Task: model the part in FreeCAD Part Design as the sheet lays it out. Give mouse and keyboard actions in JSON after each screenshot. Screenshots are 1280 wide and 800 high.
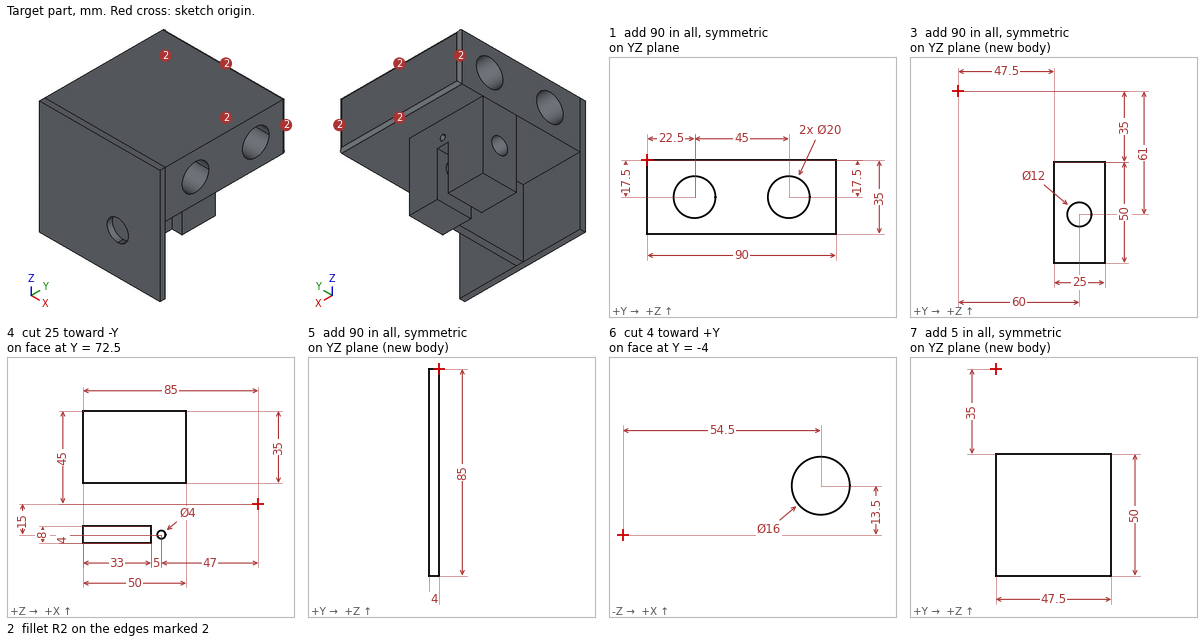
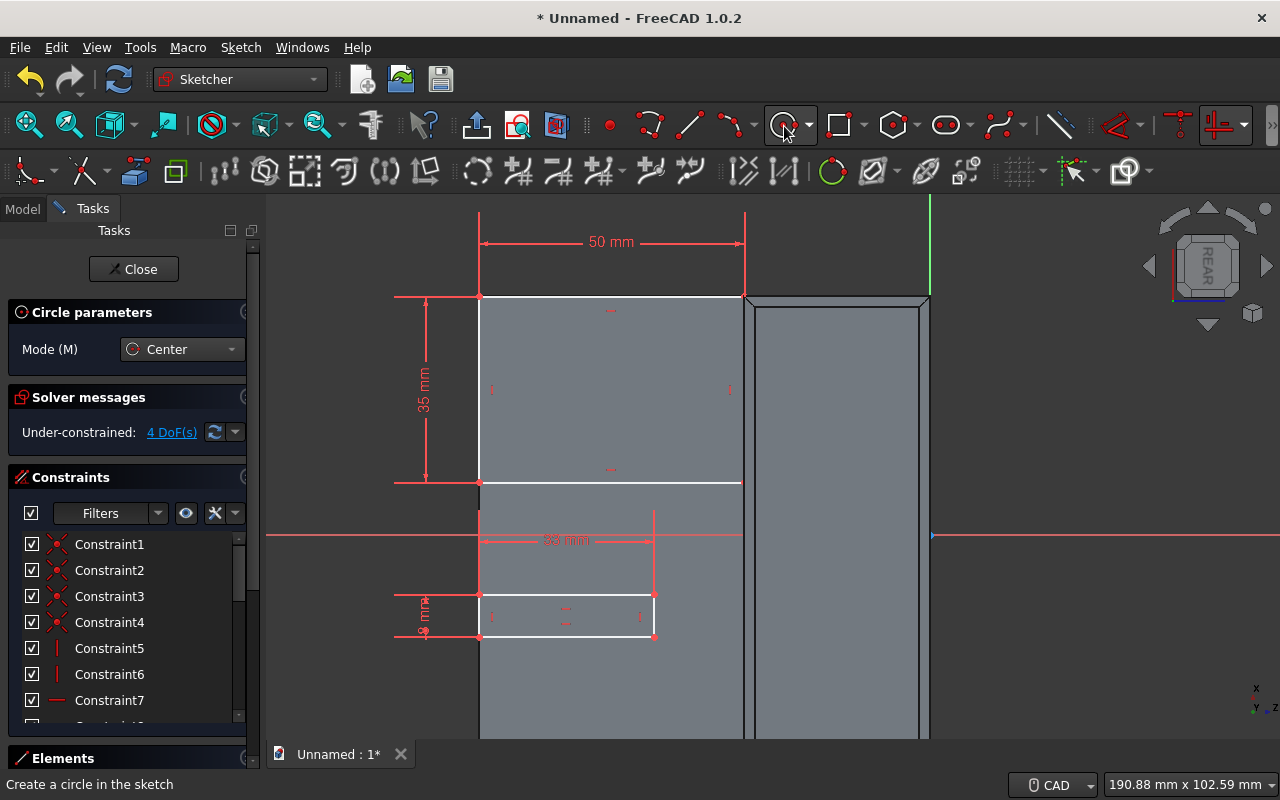
{"action": "scroll", "coordinate": [680, 615], "scroll_direction": "up", "scroll_amount": 4}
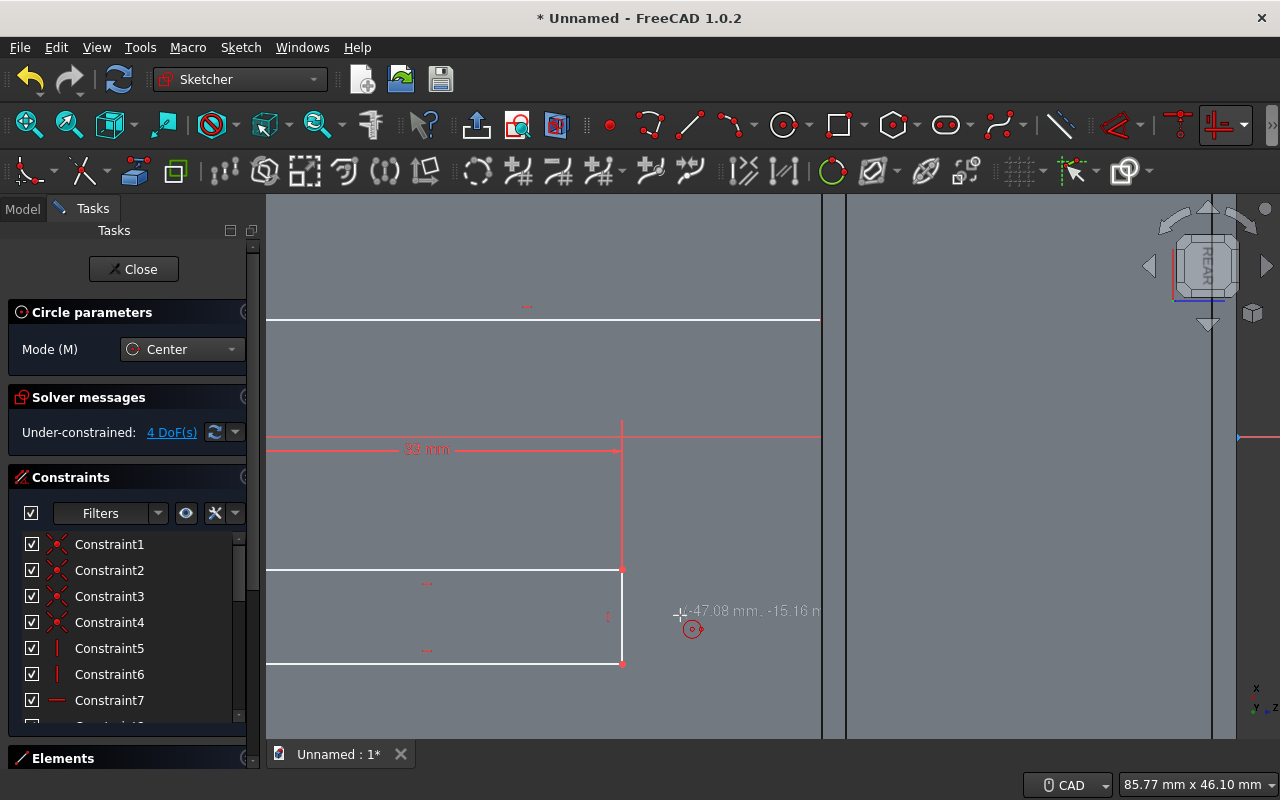
{"action": "left_click", "coordinate": [680, 614]}
{"action": "mouse_move", "coordinate": [697, 598]}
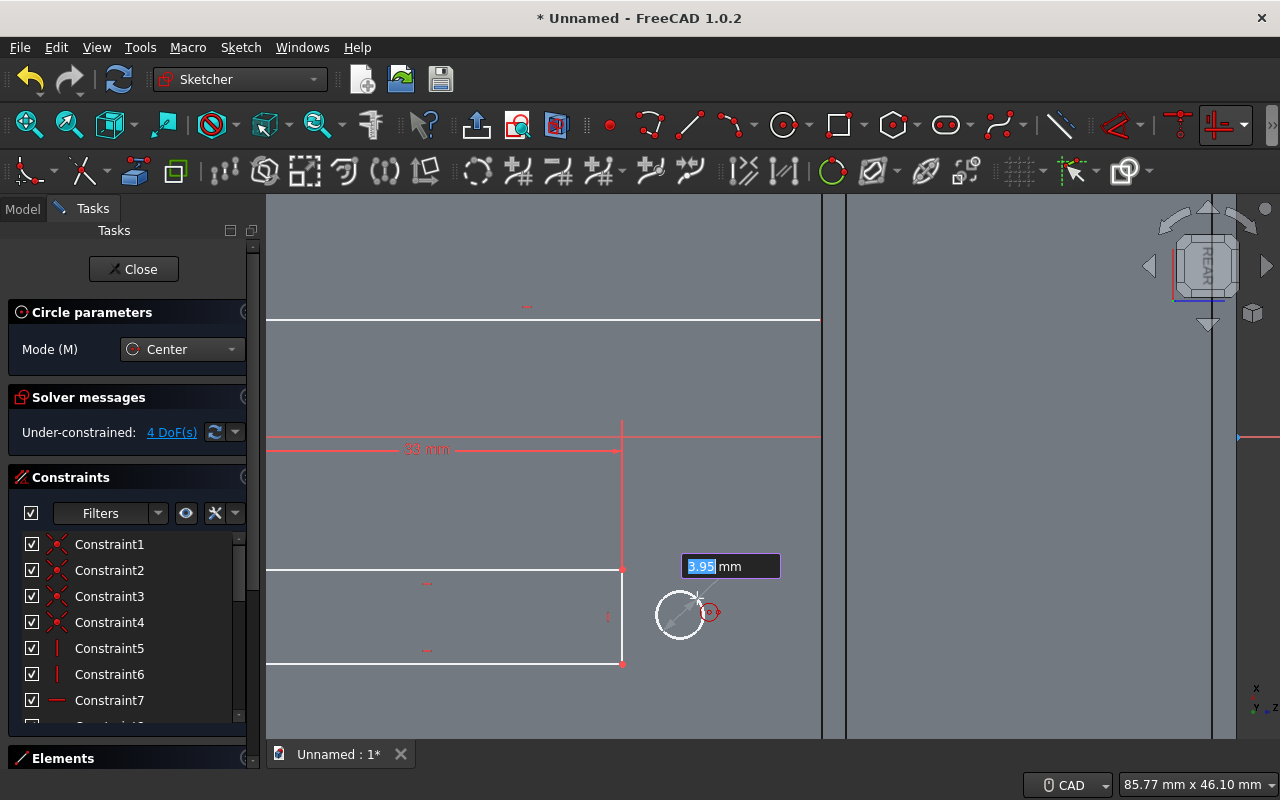
{"action": "type", "text": "4"}
{"action": "key", "text": "Return"}
{"action": "key", "text": "Escape"}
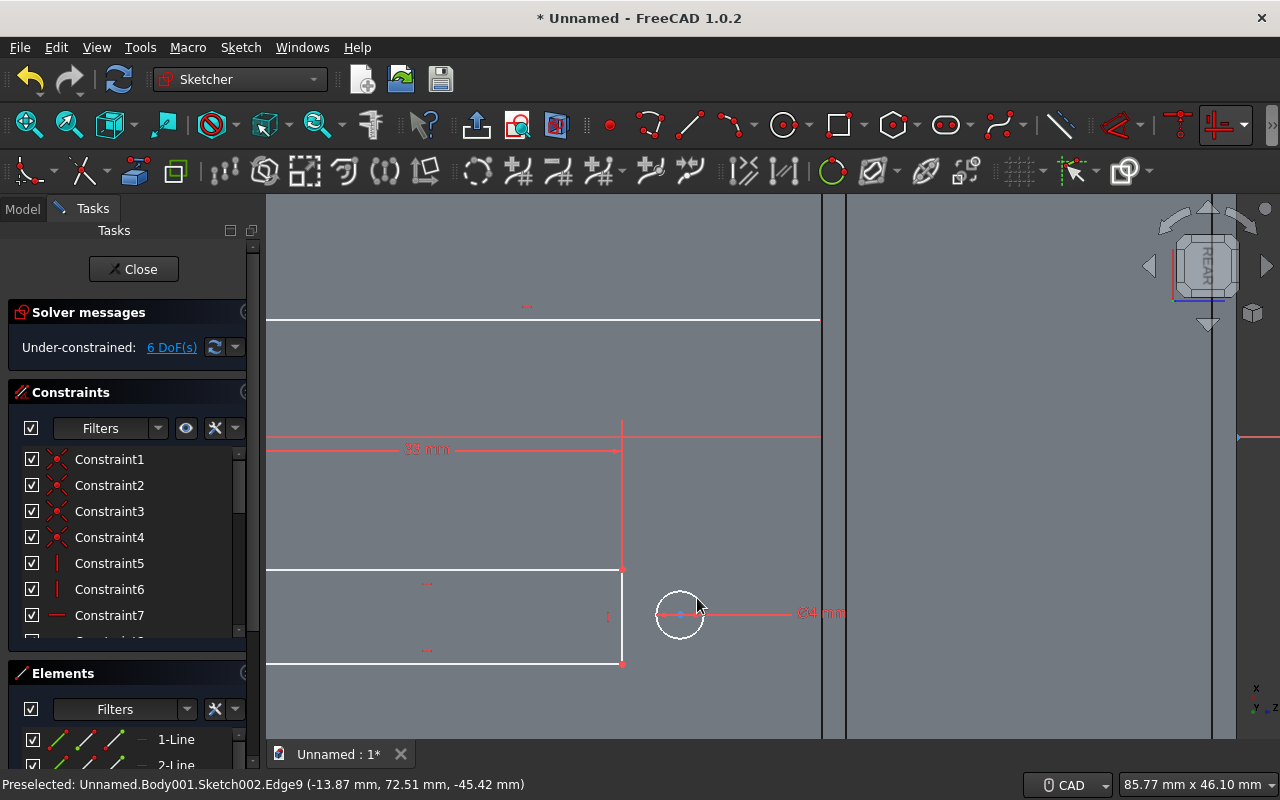
{"action": "key", "text": "d"}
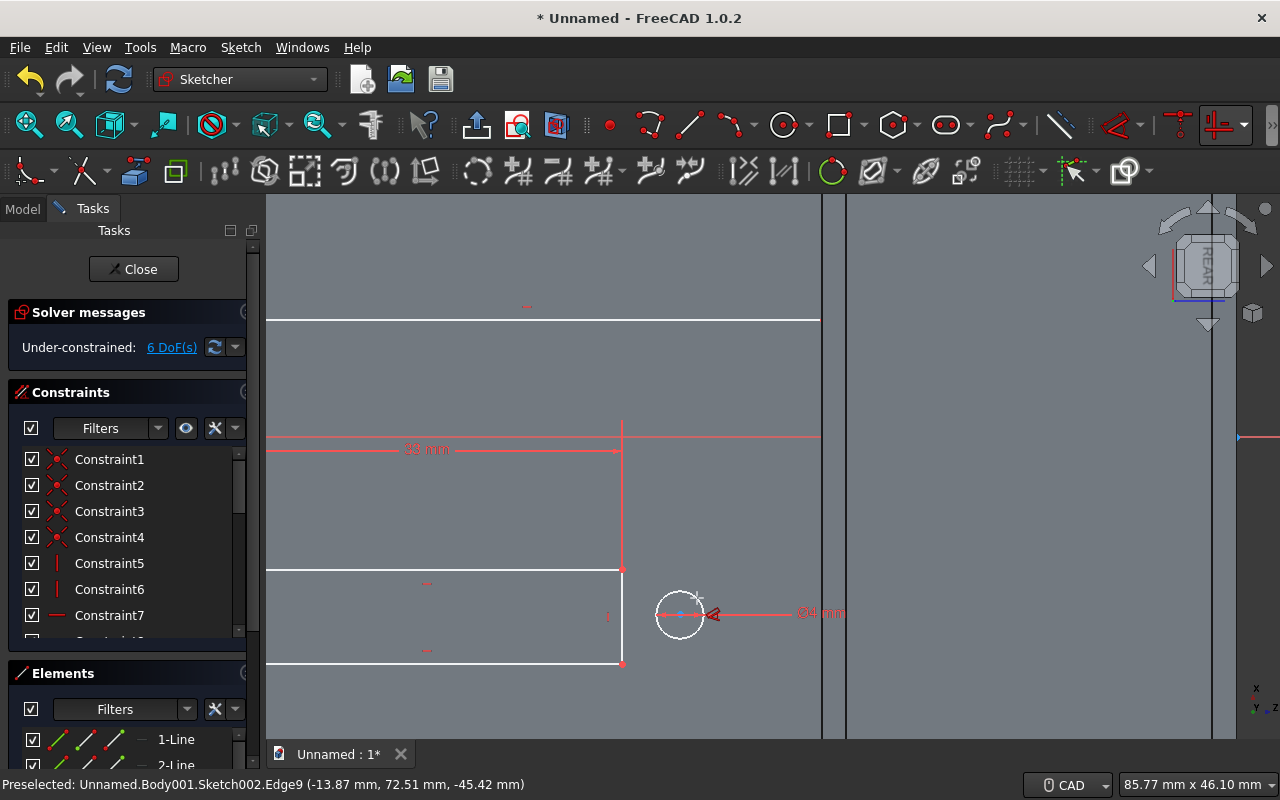
{"action": "left_click", "coordinate": [680, 615]}
{"action": "left_click", "coordinate": [897, 649]}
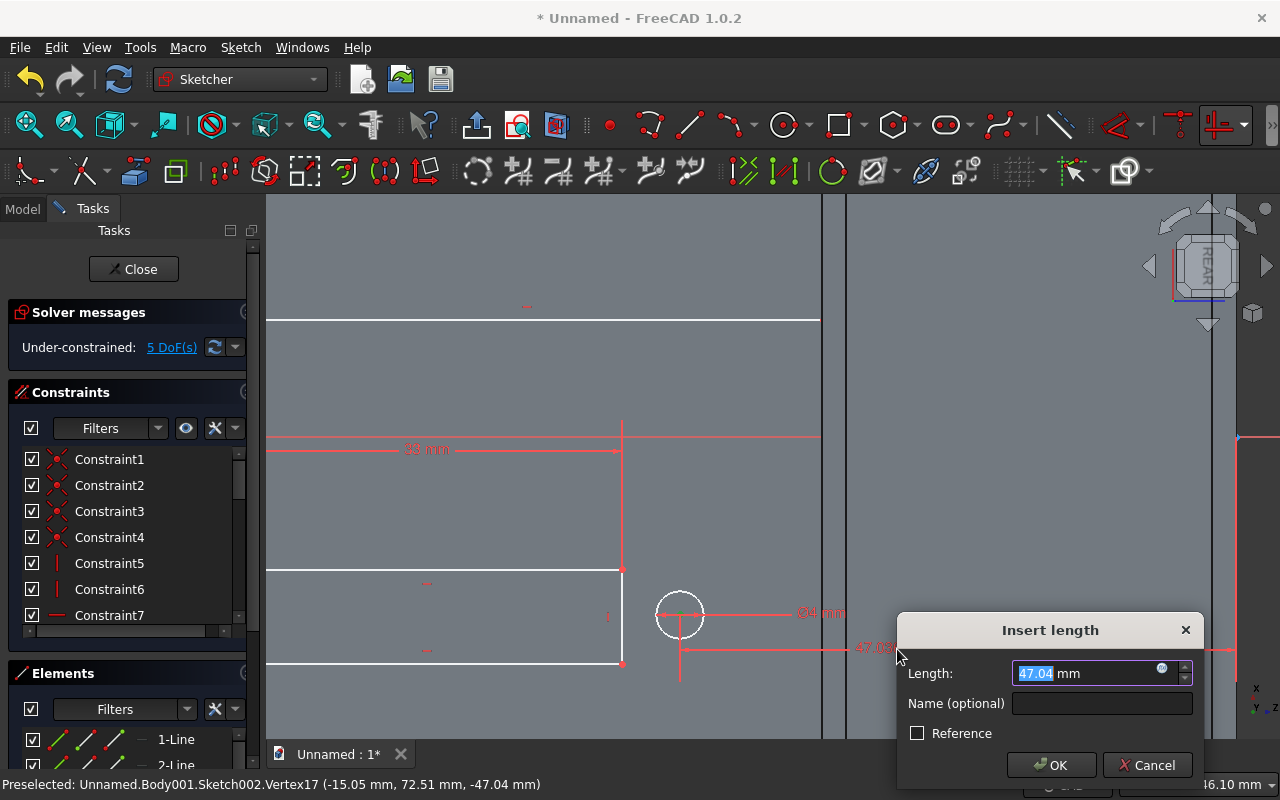
{"action": "type", "text": "47"}
{"action": "key", "text": "Return"}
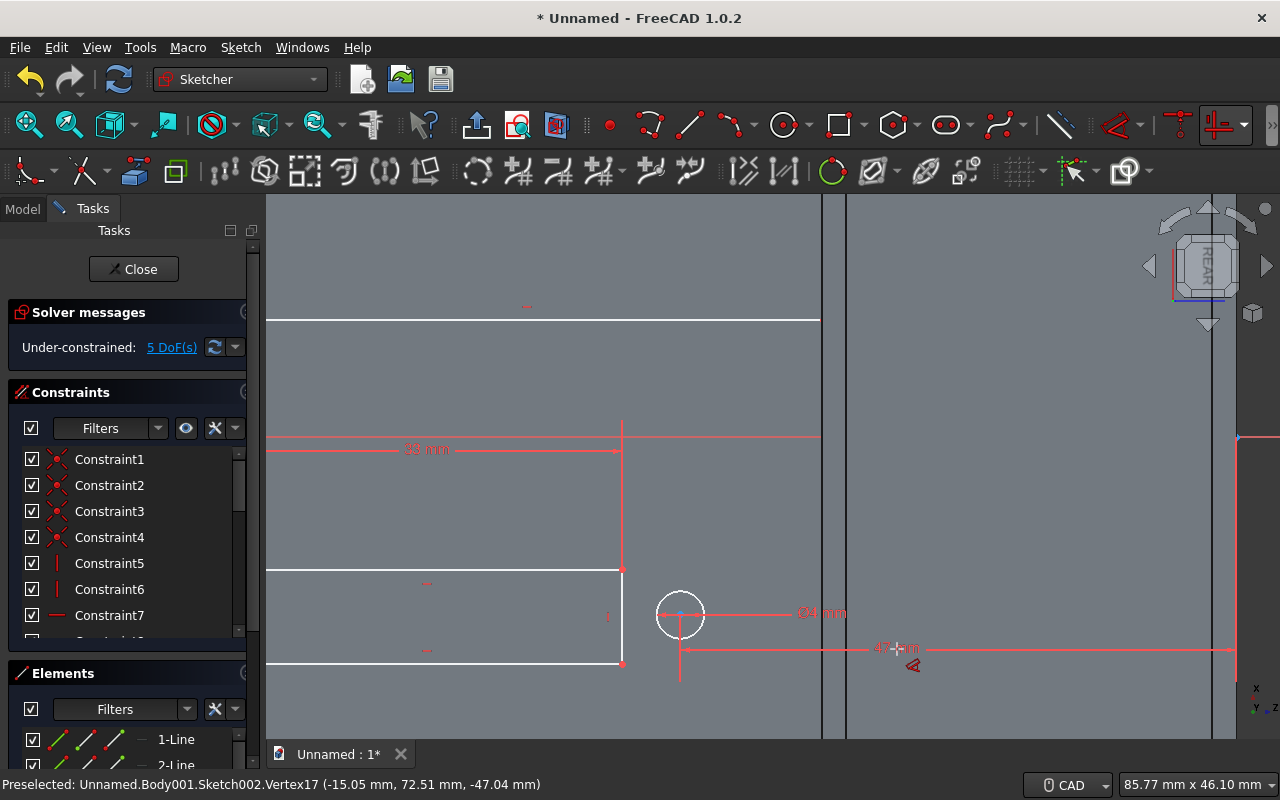
{"action": "left_click", "coordinate": [680, 615]}
{"action": "left_click", "coordinate": [646, 526]}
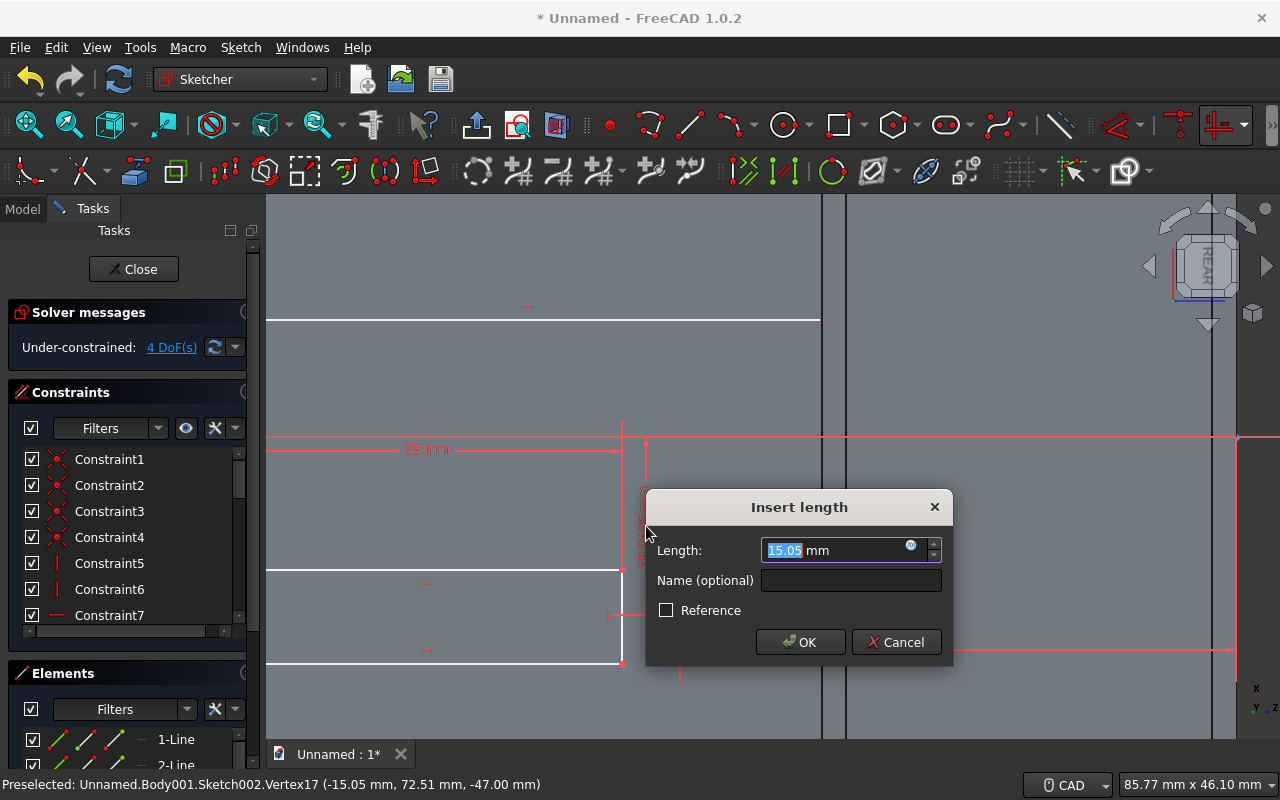
{"action": "type", "text": "15"}
{"action": "key", "text": "Return"}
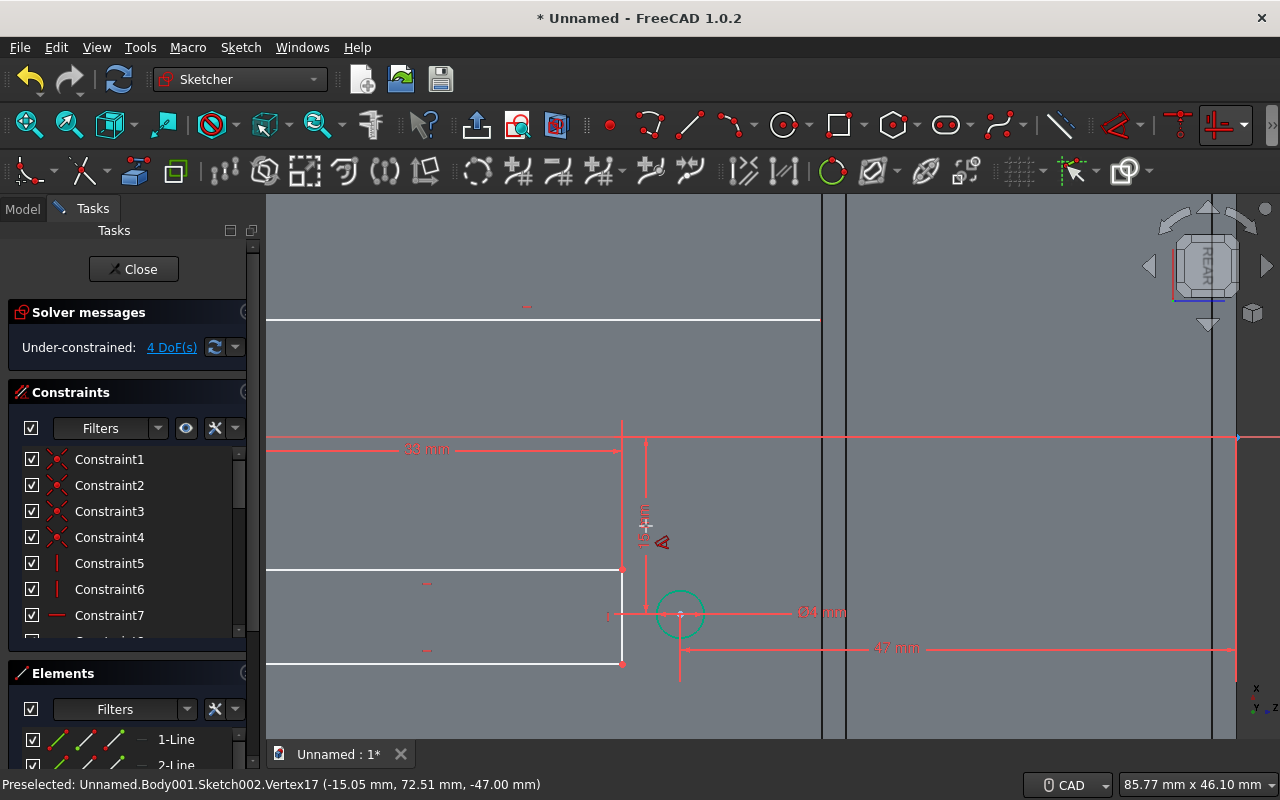
{"action": "left_click", "coordinate": [622, 664]}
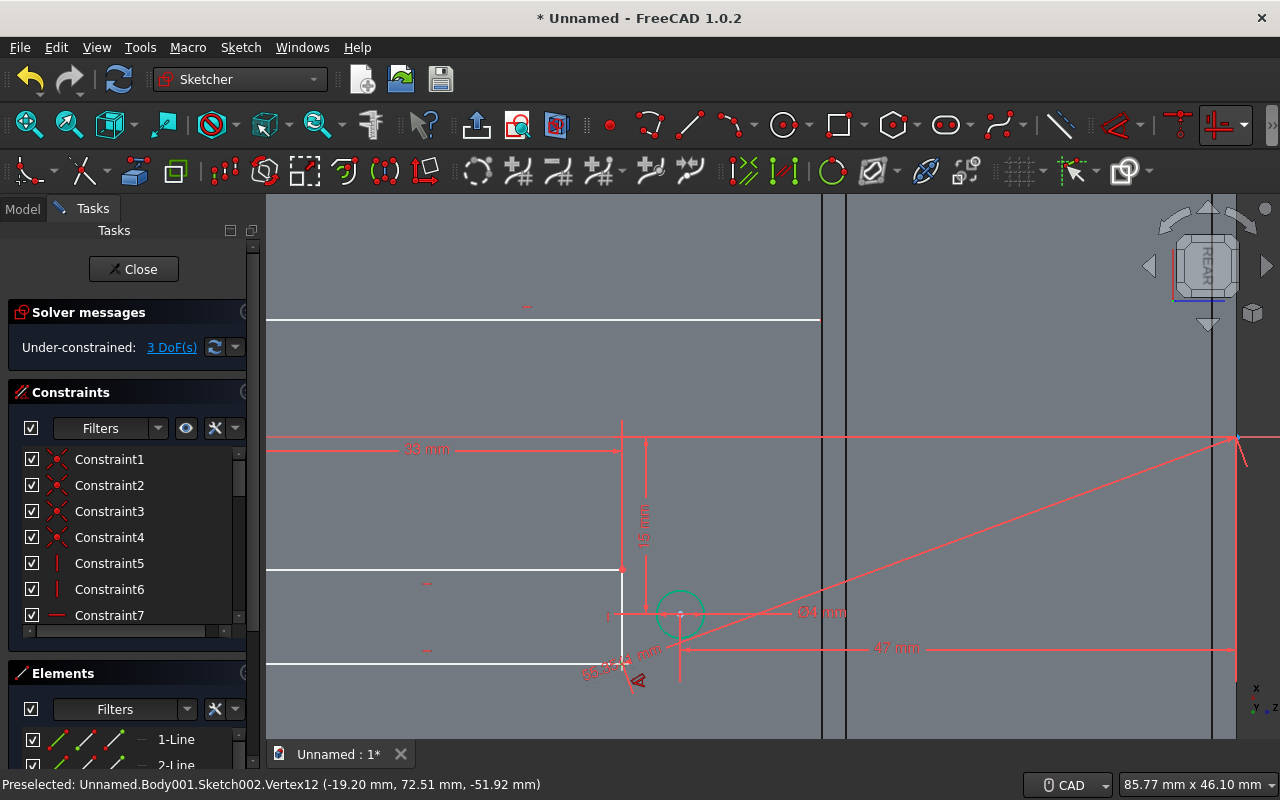
{"action": "left_click", "coordinate": [680, 614]}
{"action": "left_click", "coordinate": [651, 698]}